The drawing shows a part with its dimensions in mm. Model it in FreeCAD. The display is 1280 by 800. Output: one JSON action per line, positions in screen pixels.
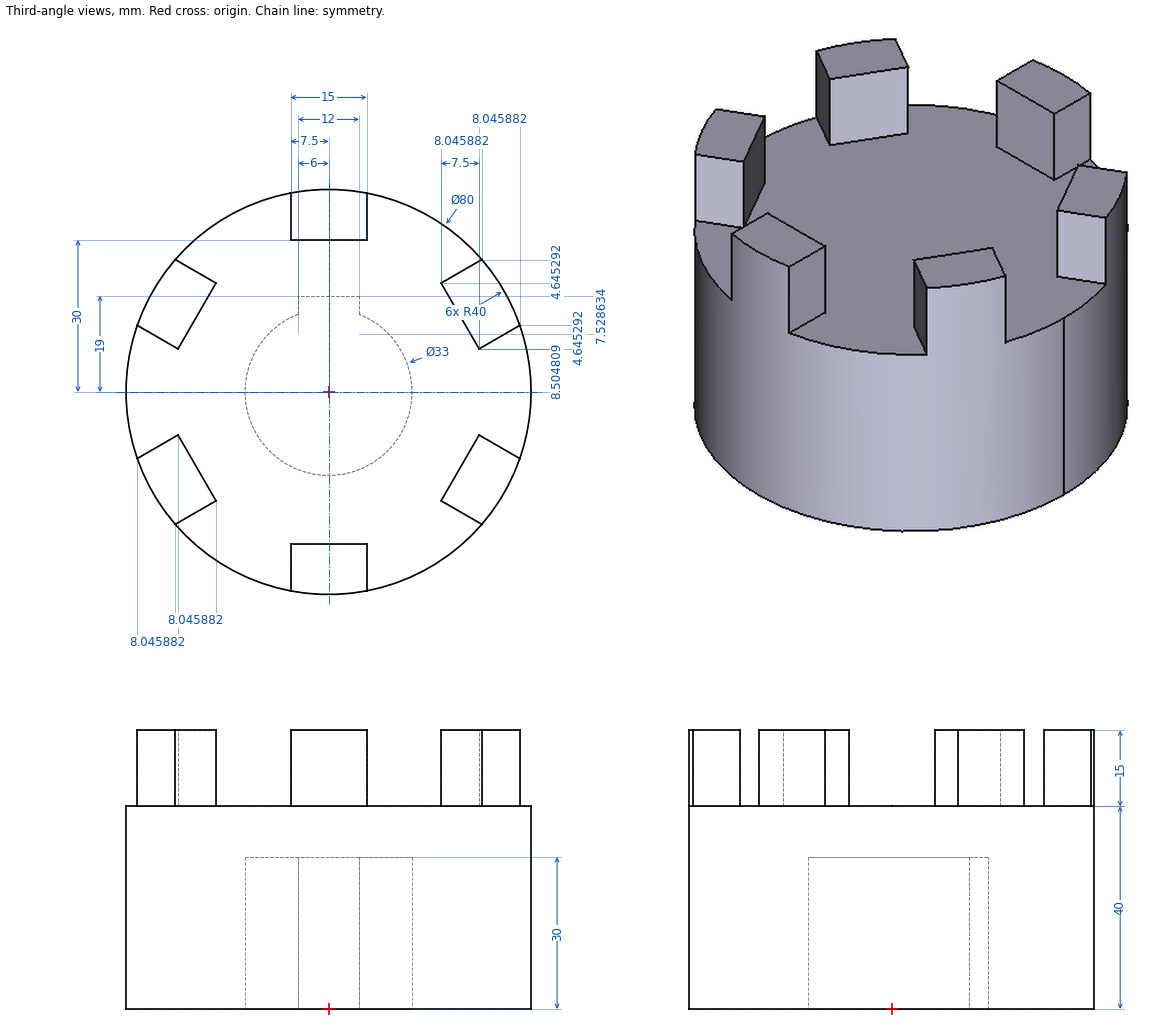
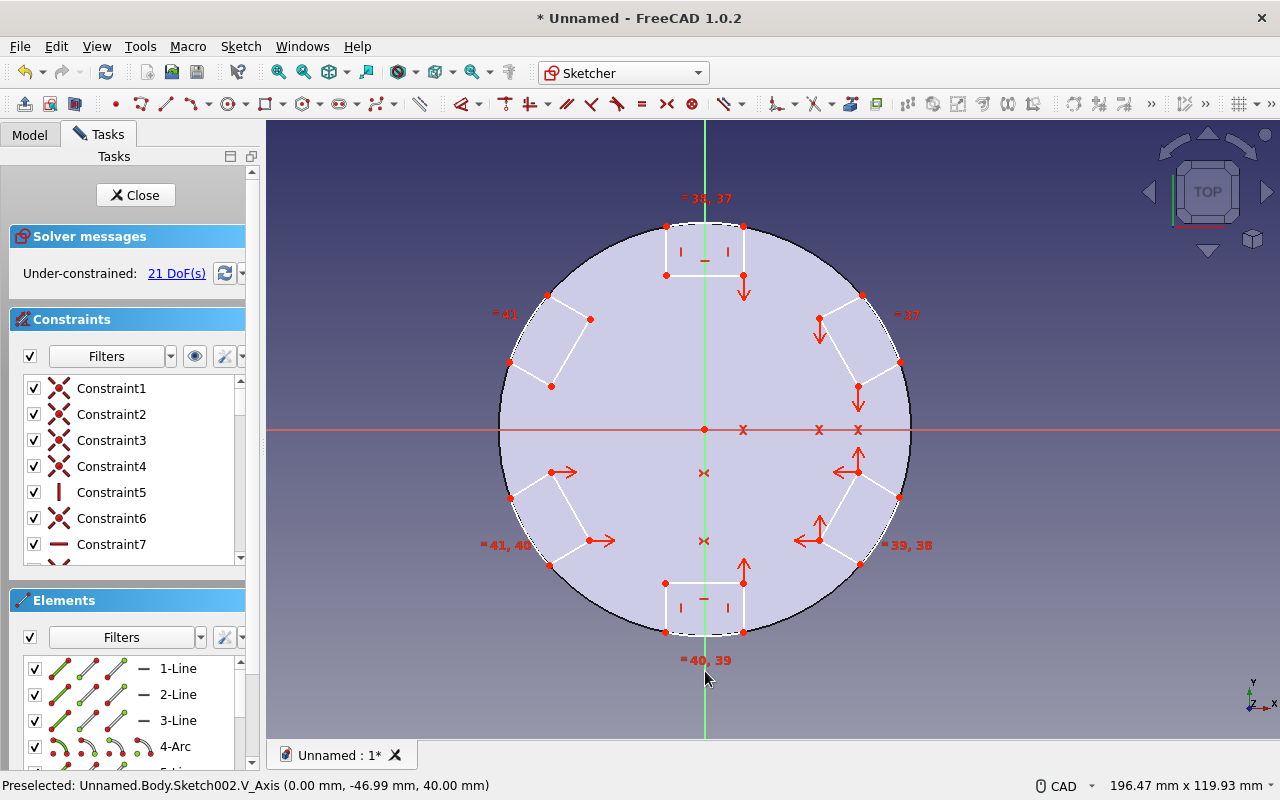
{"action": "left_click", "coordinate": [858, 387]}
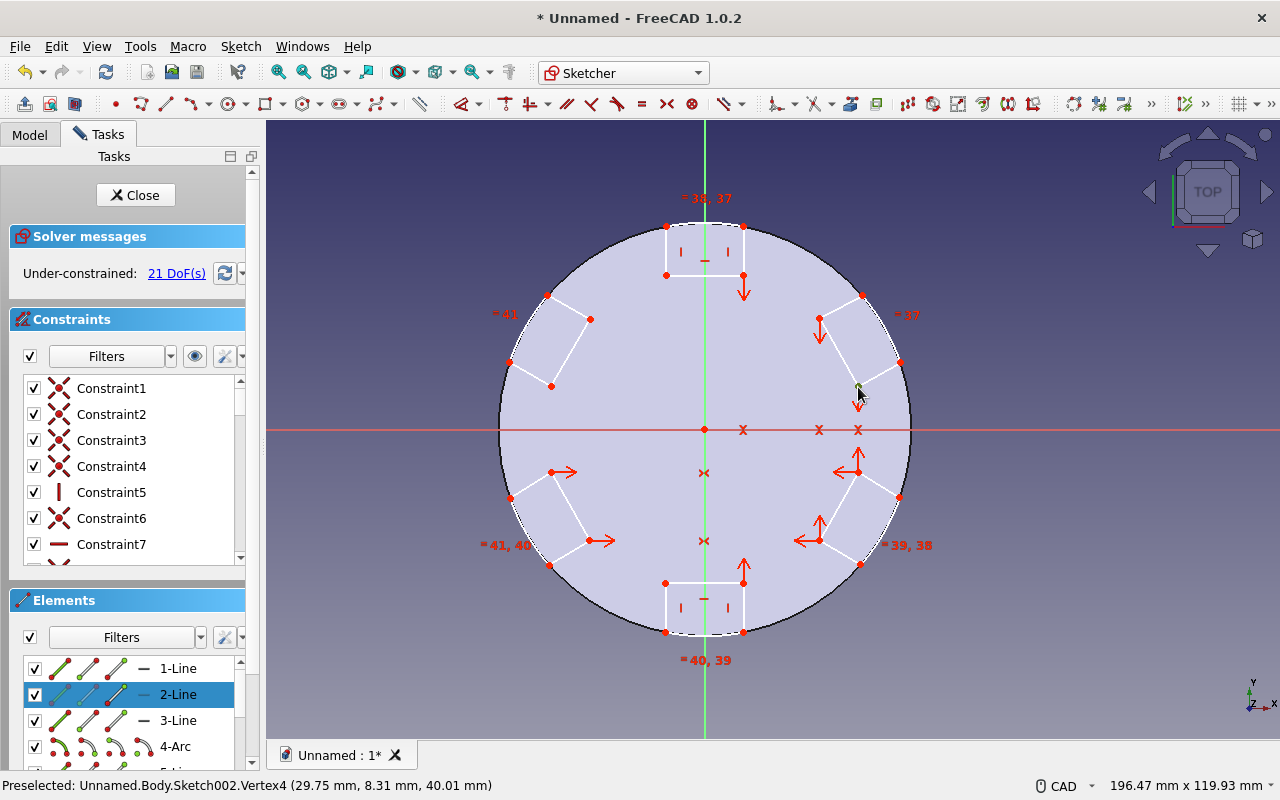
{"action": "left_click", "coordinate": [551, 386]}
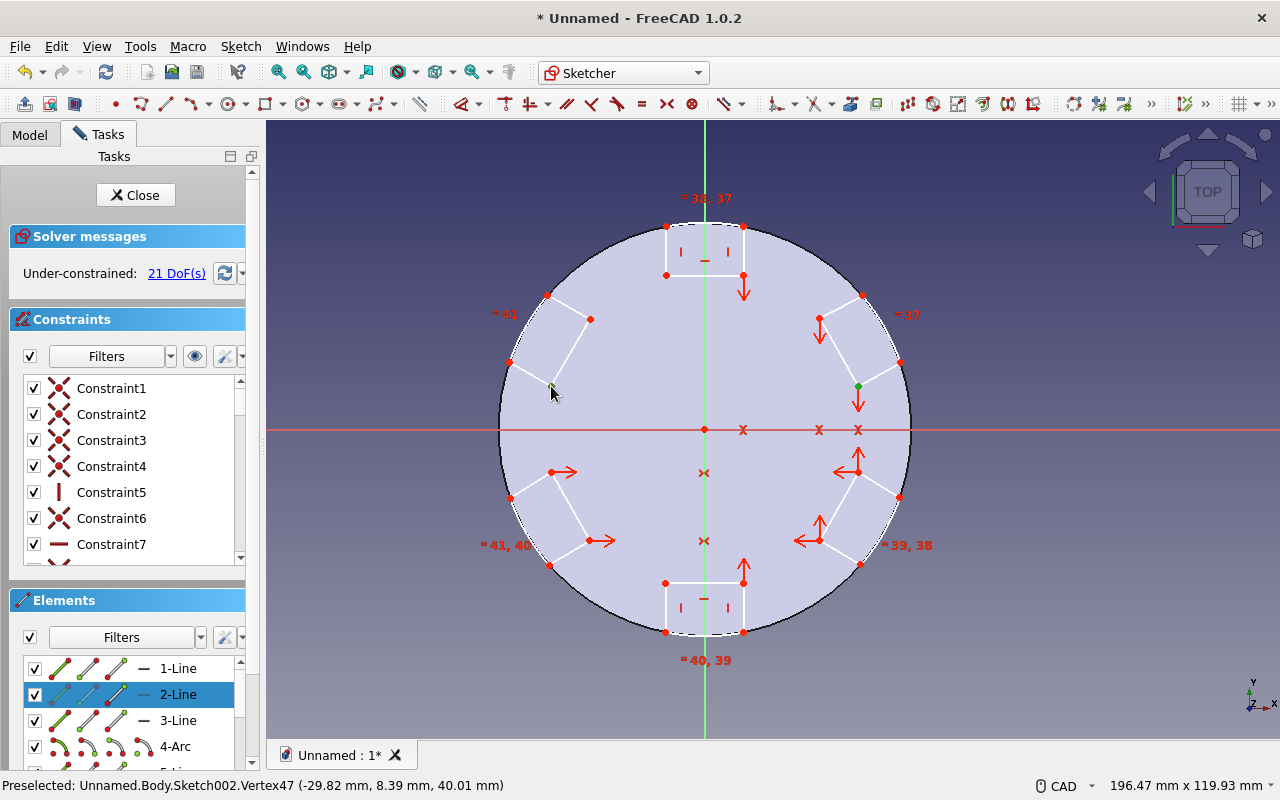
{"action": "left_click", "coordinate": [705, 671]}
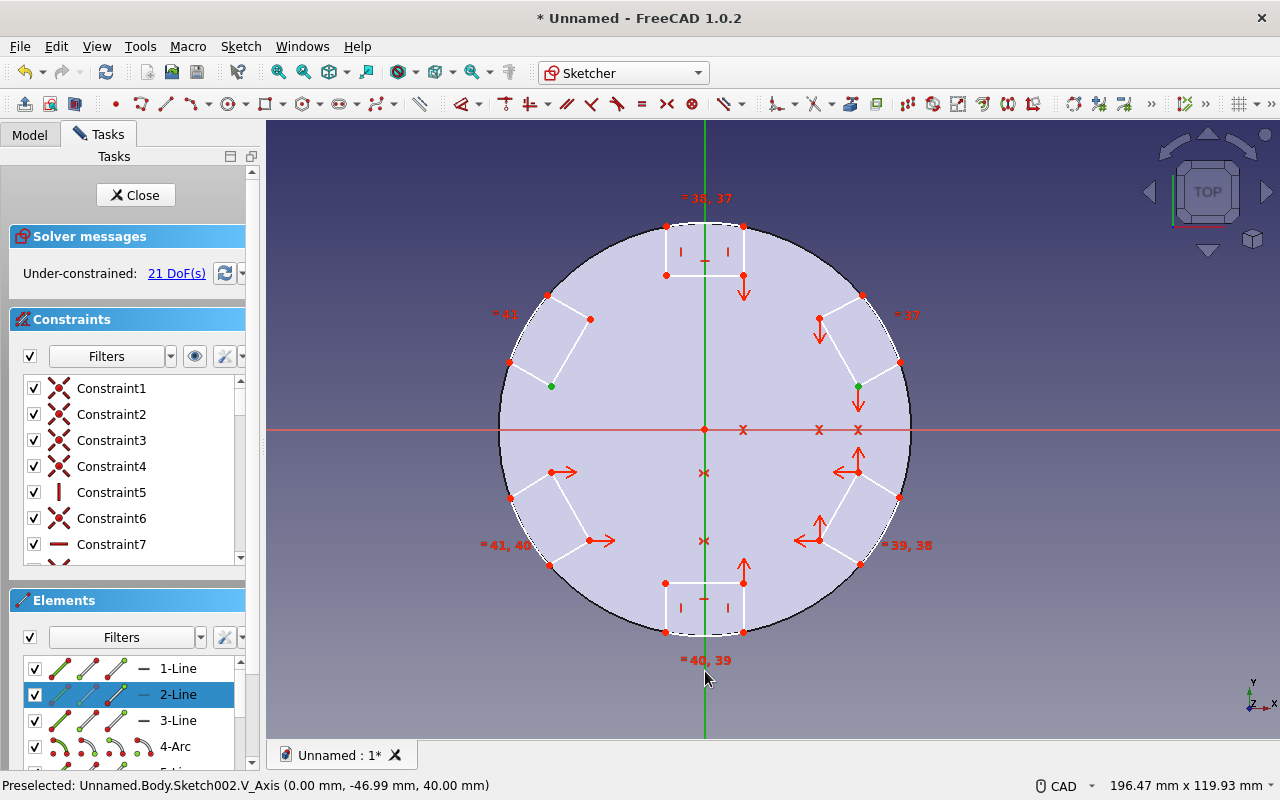
{"action": "key", "text": "s"}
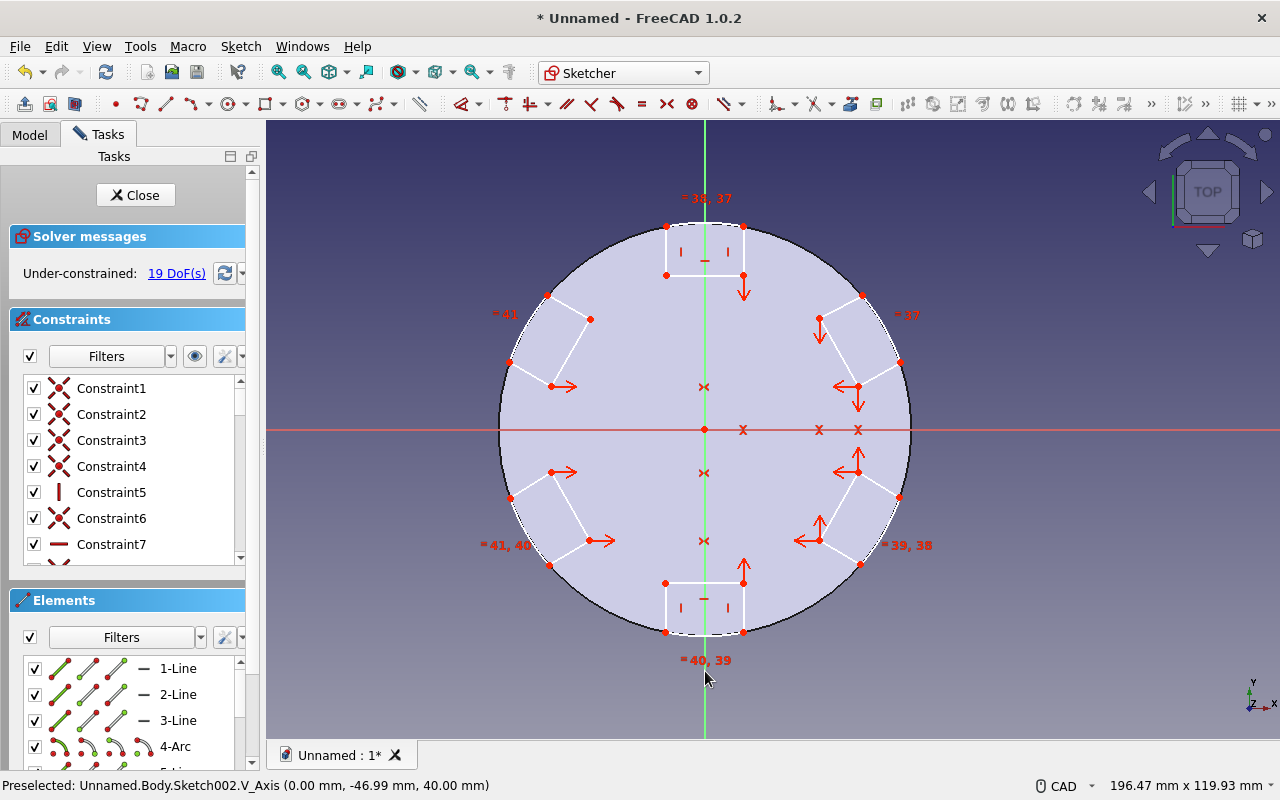
{"action": "left_click", "coordinate": [820, 318]}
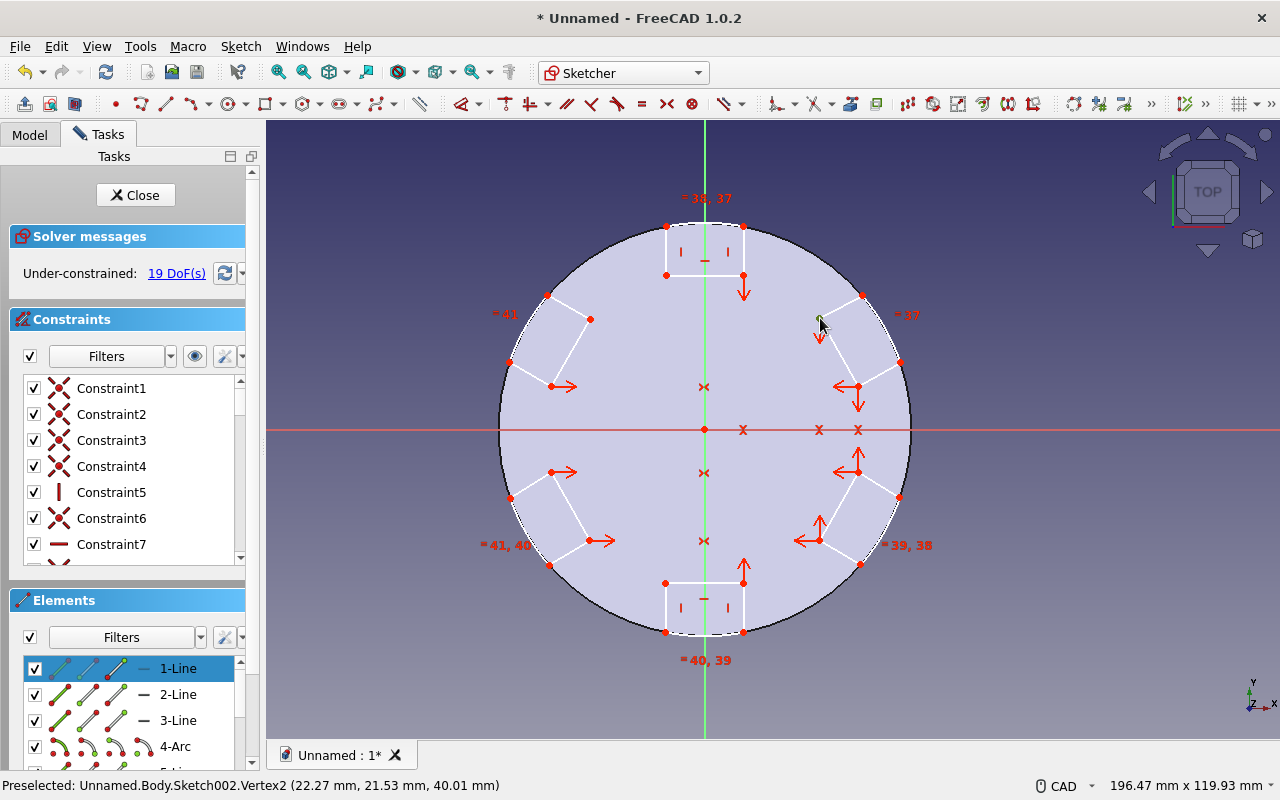
{"action": "left_click", "coordinate": [590, 319]}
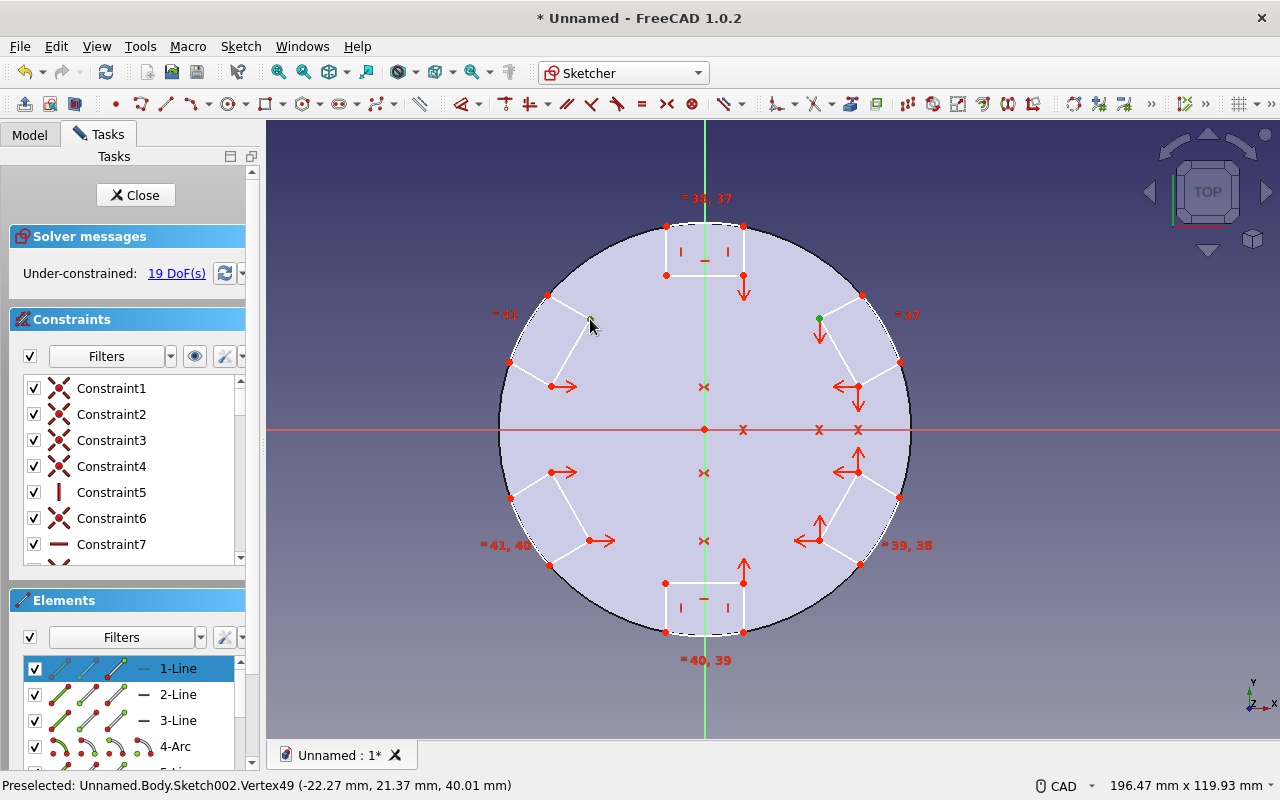
{"action": "left_click", "coordinate": [705, 671]}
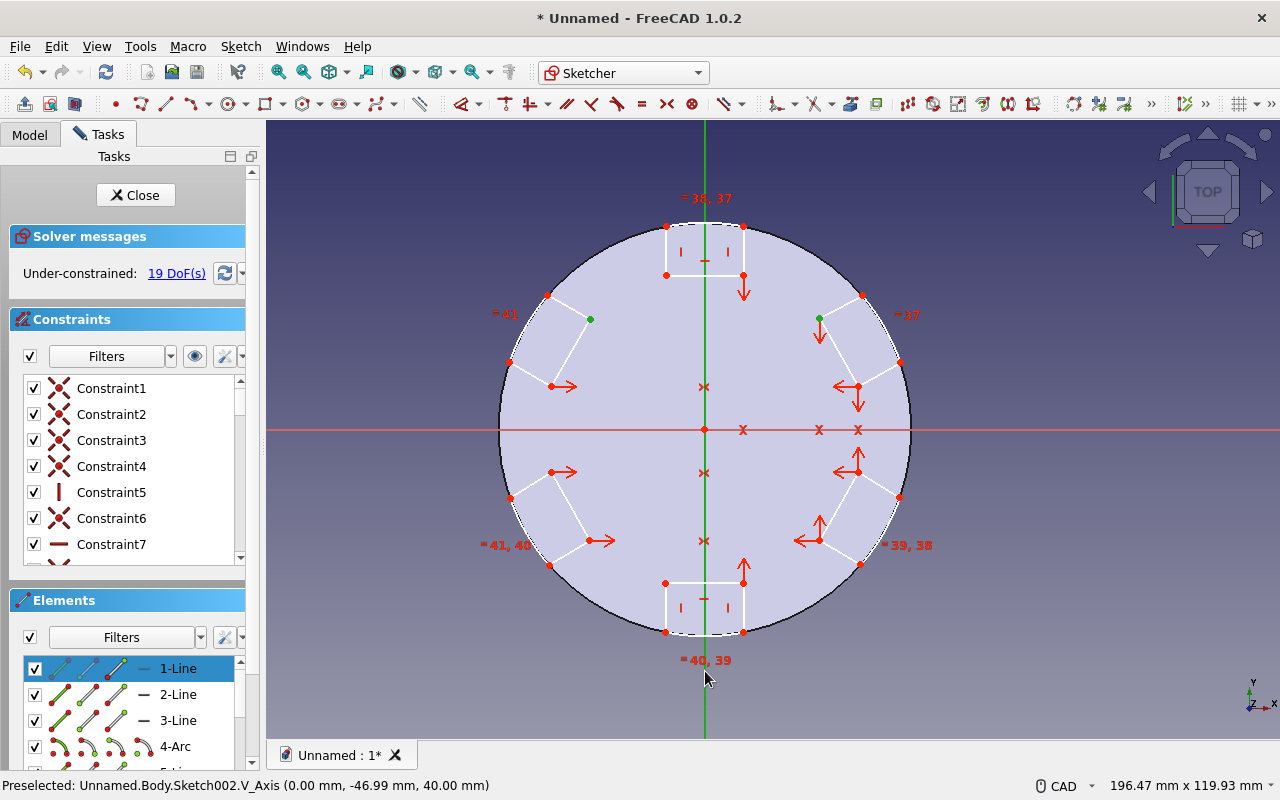
{"action": "left_click", "coordinate": [667, 104]}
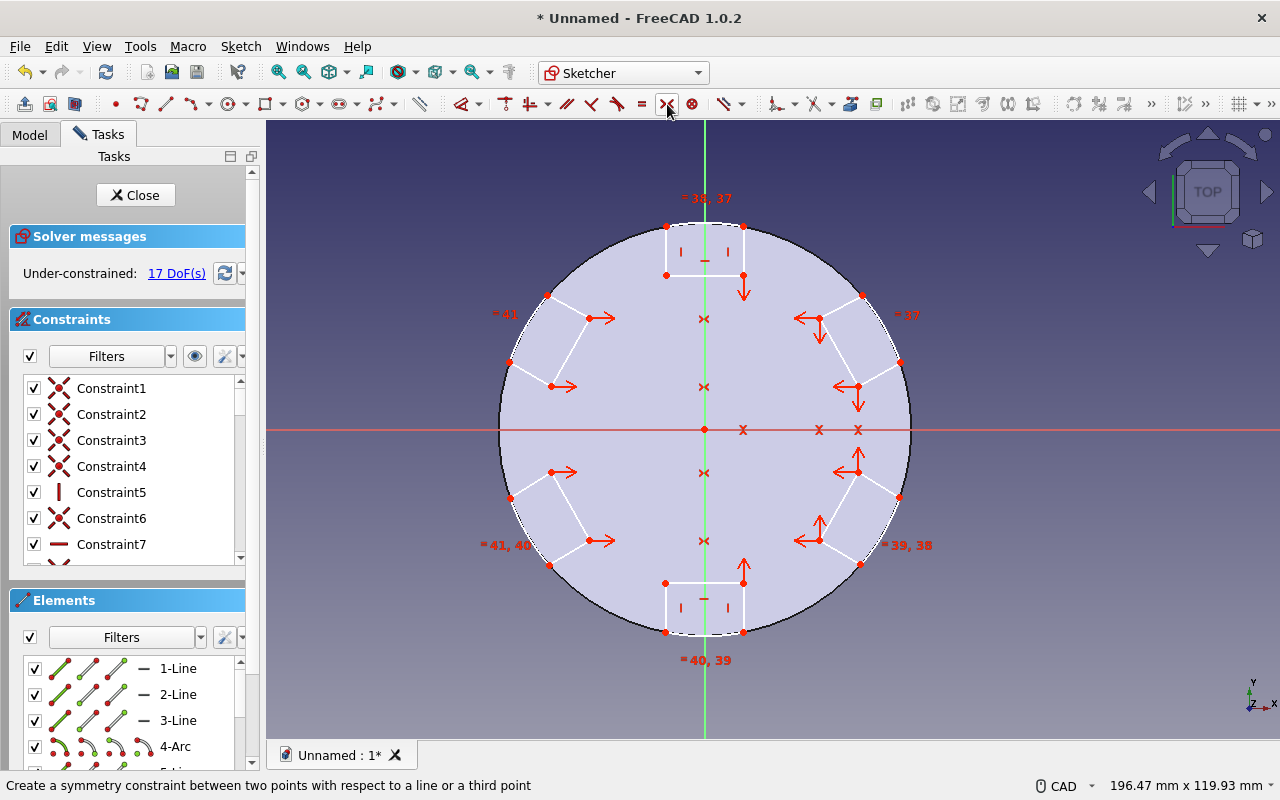
{"action": "left_click", "coordinate": [460, 104]}